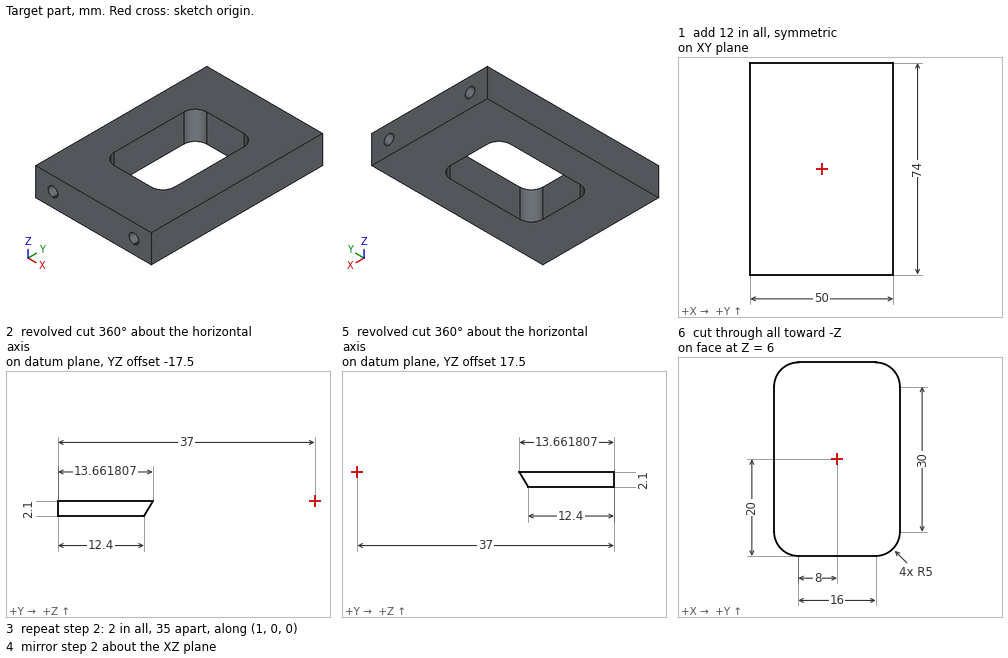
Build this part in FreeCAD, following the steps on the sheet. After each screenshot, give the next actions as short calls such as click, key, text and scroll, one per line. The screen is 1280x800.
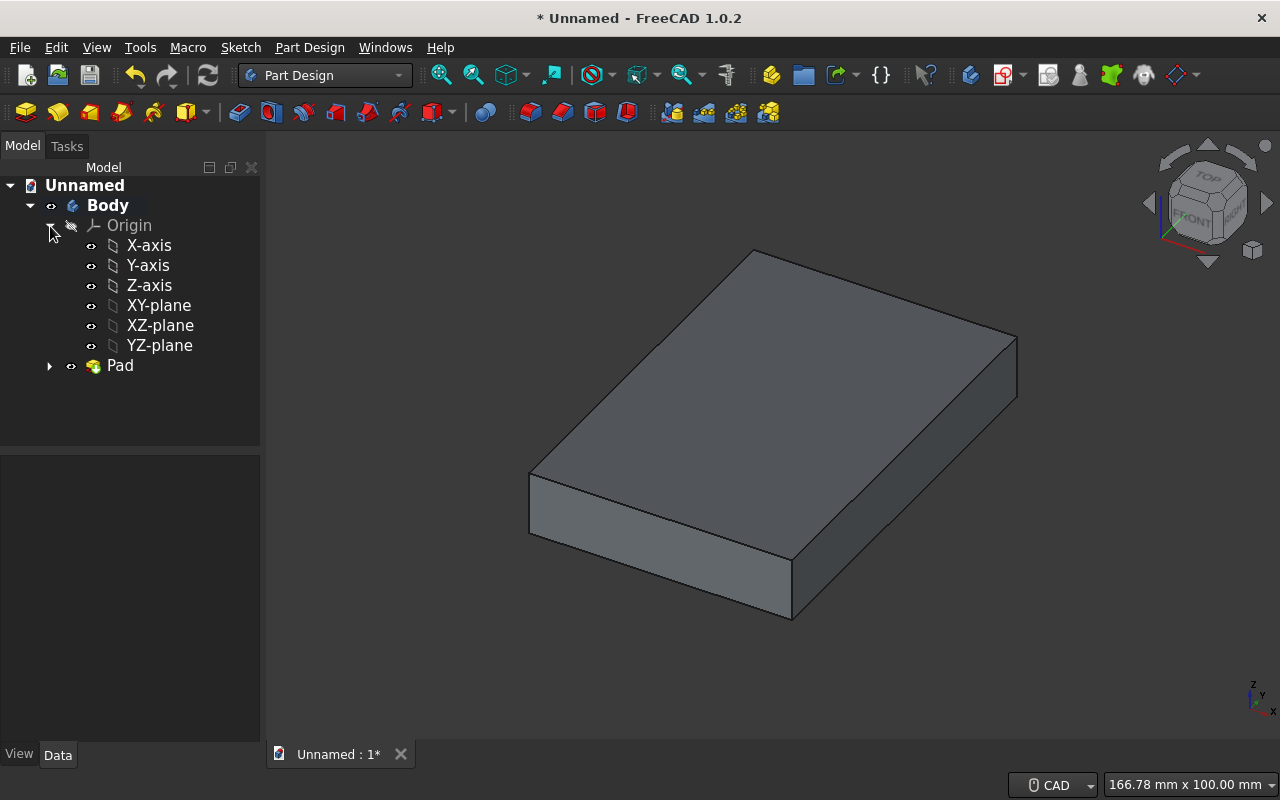
click(136, 346)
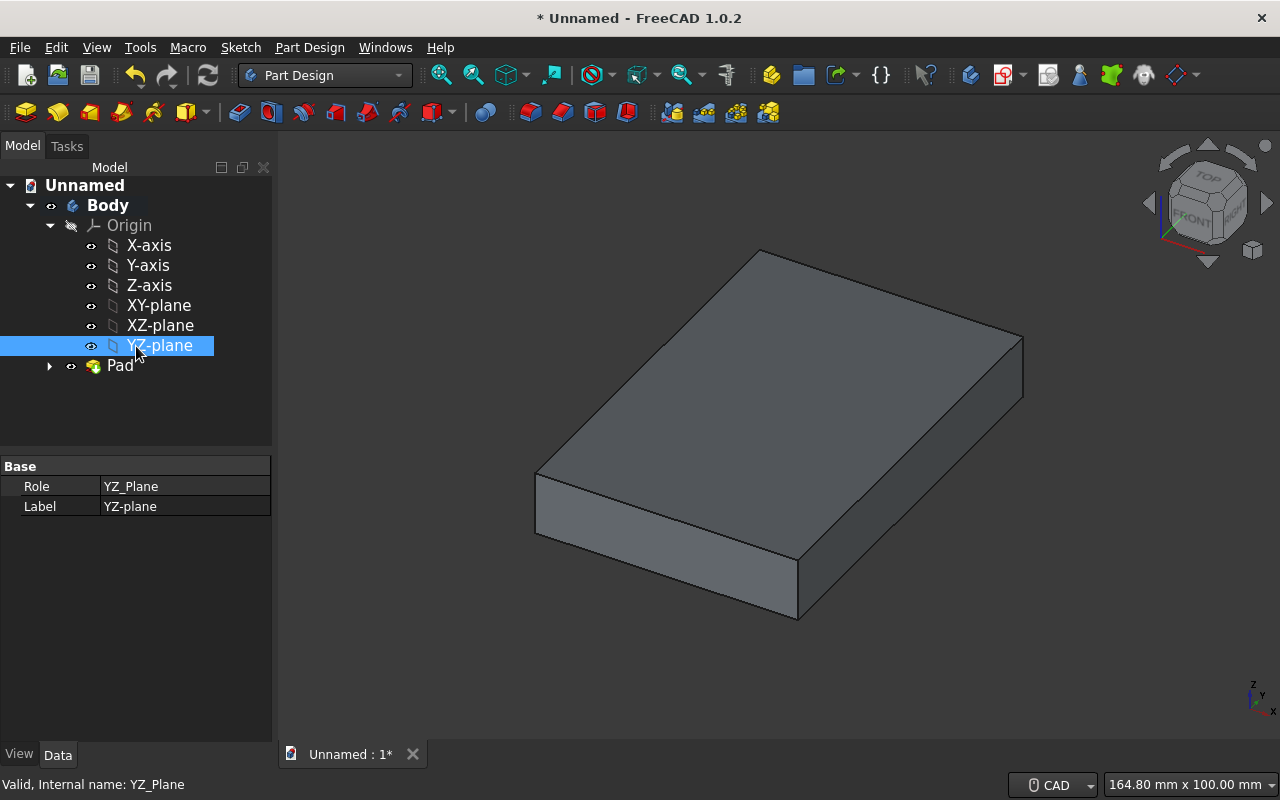
click(1176, 76)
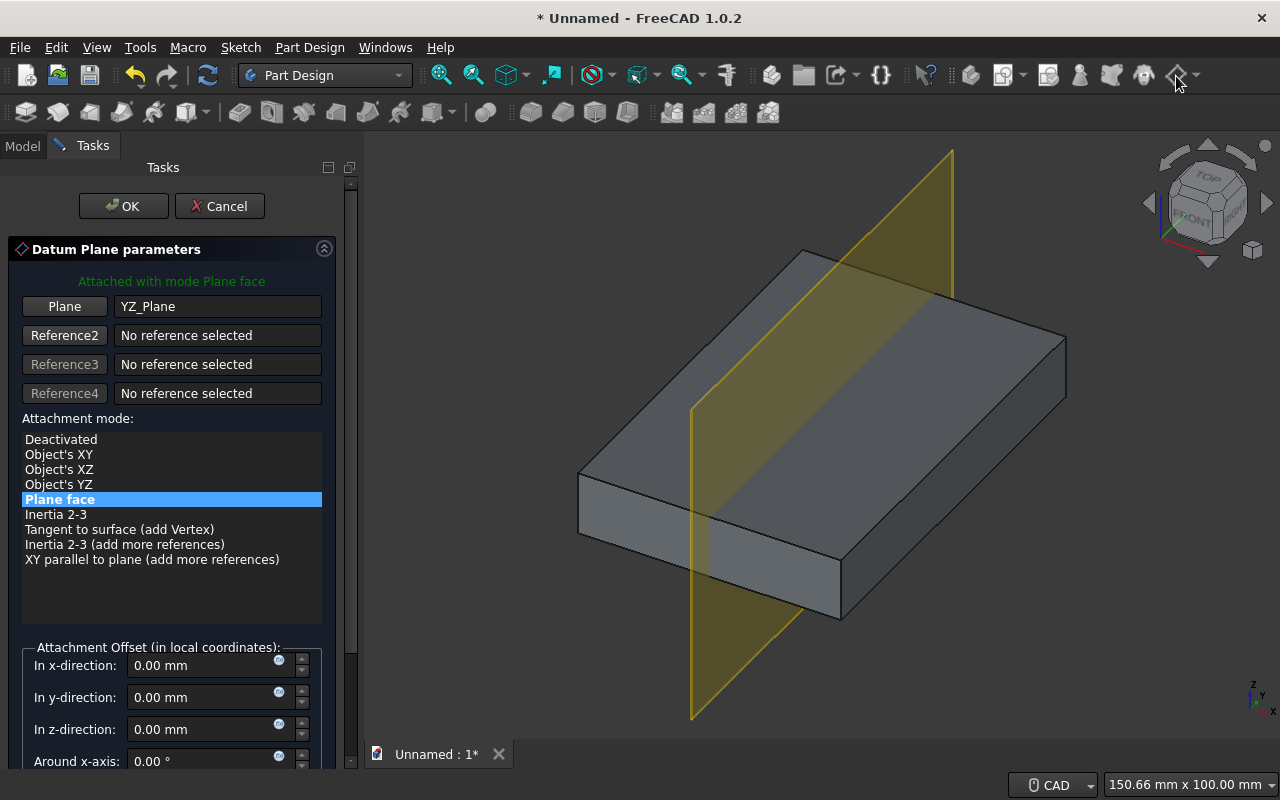
triple_click(210, 729)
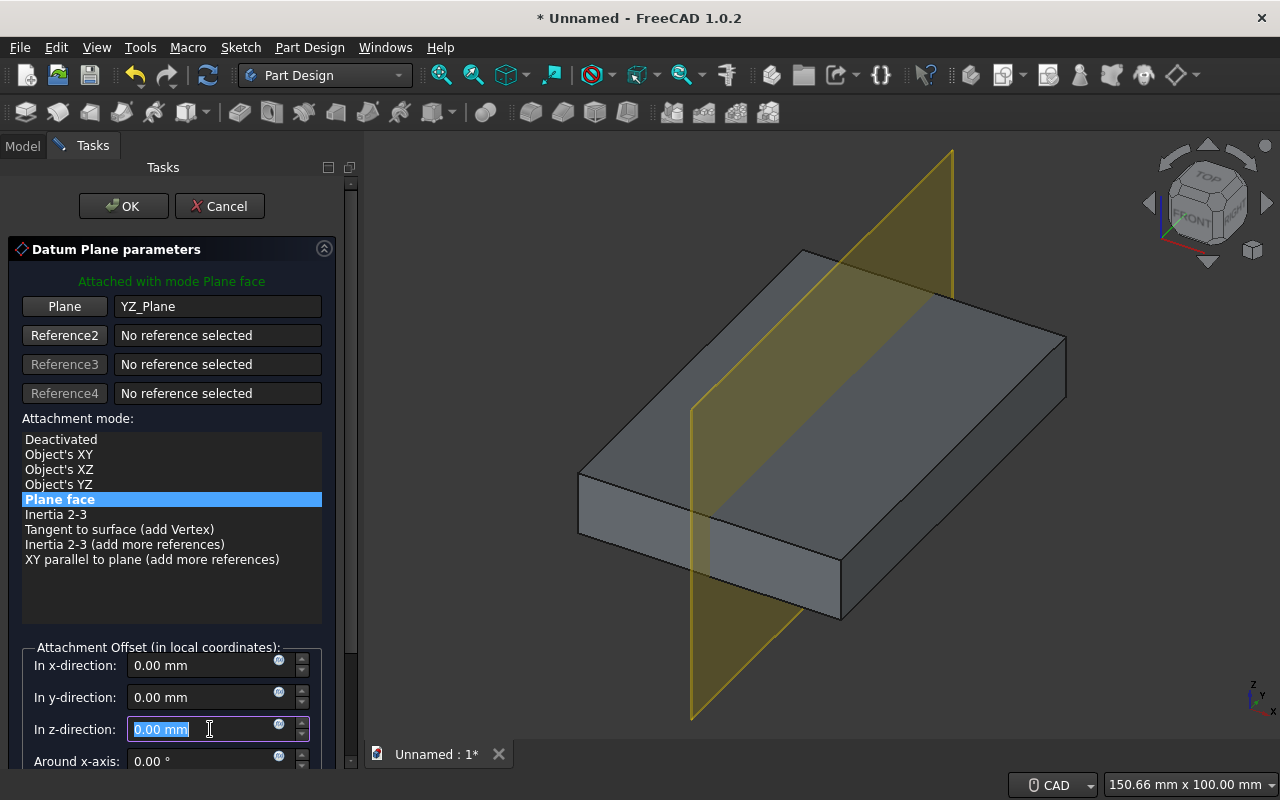
text(-17.5)
key(Tab)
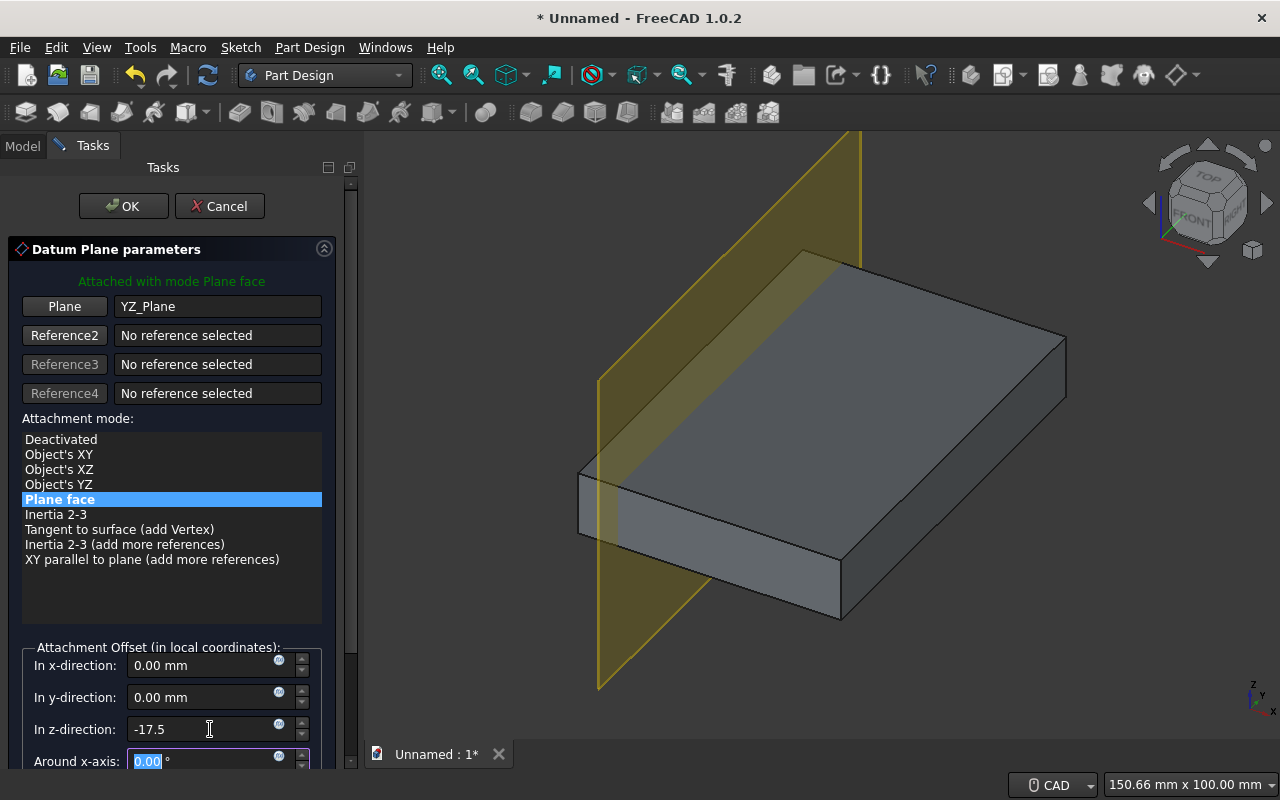
click(124, 206)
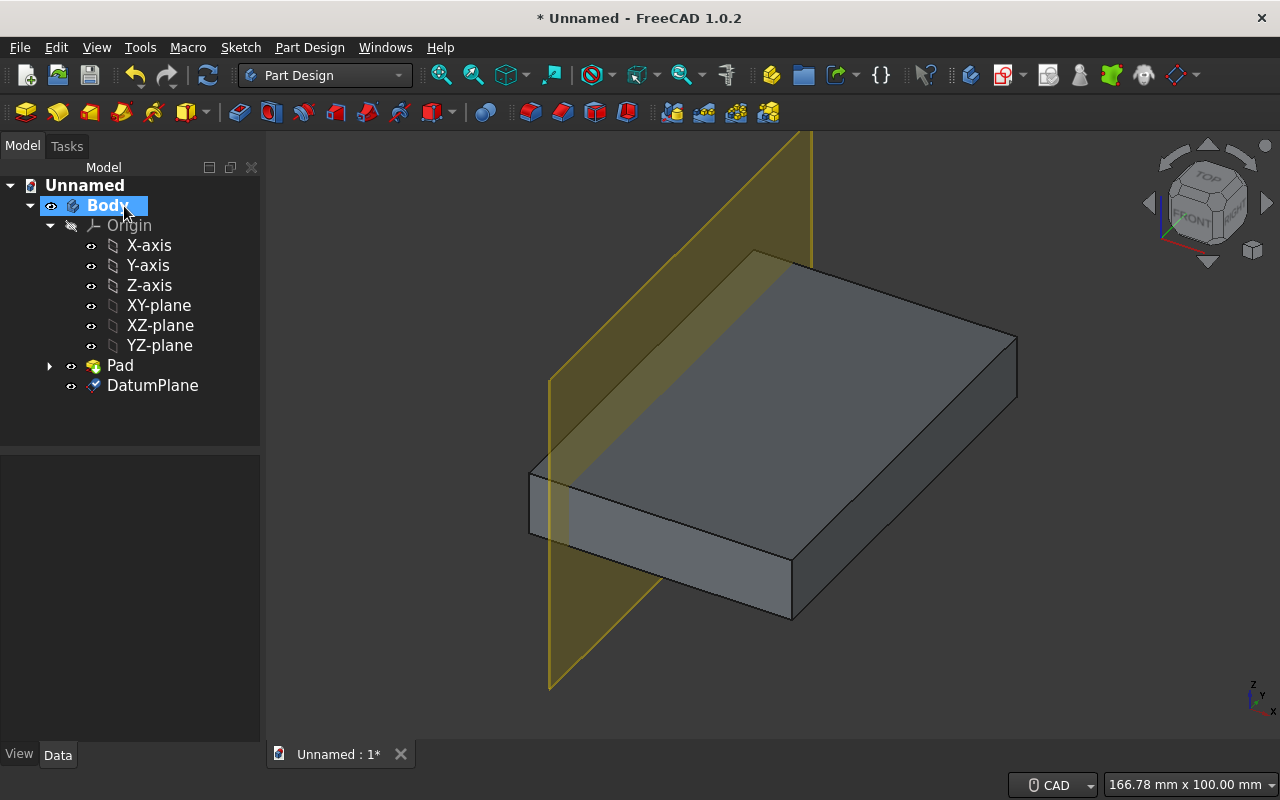
click(116, 386)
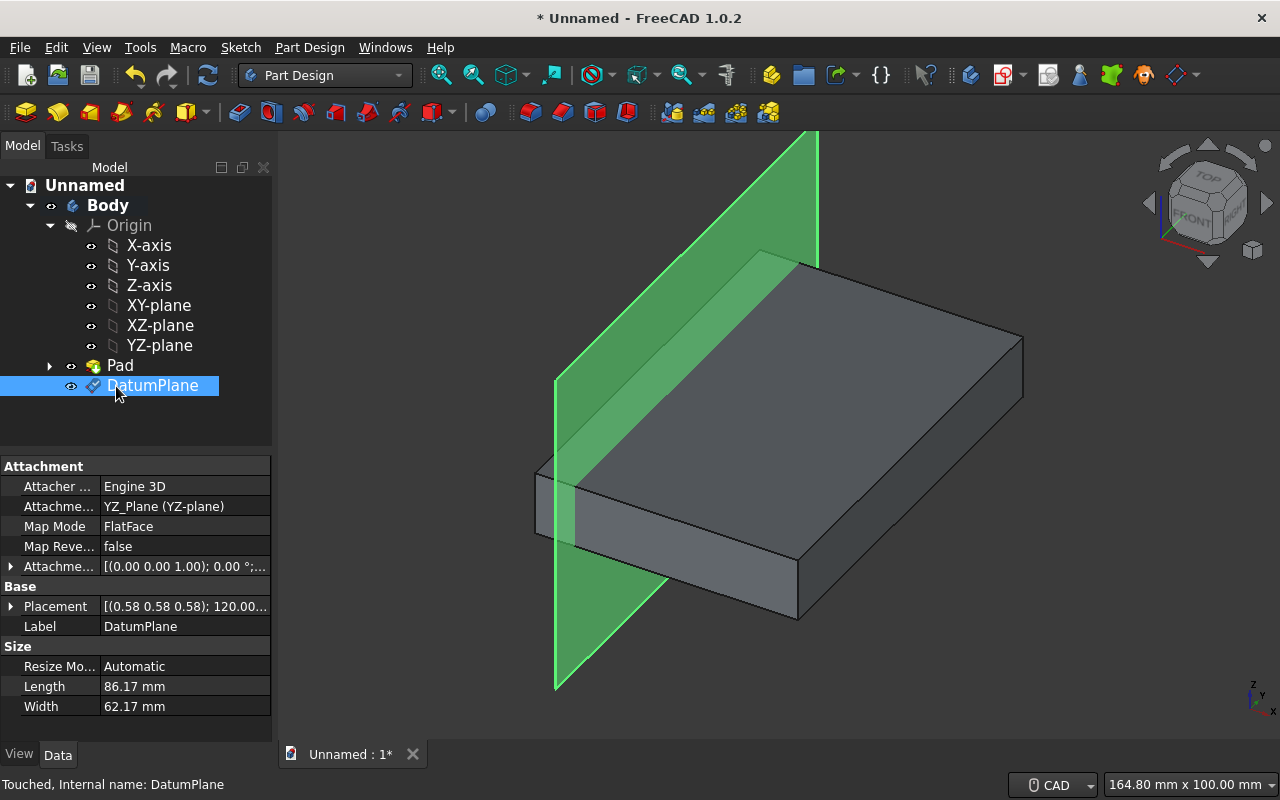
click(1004, 76)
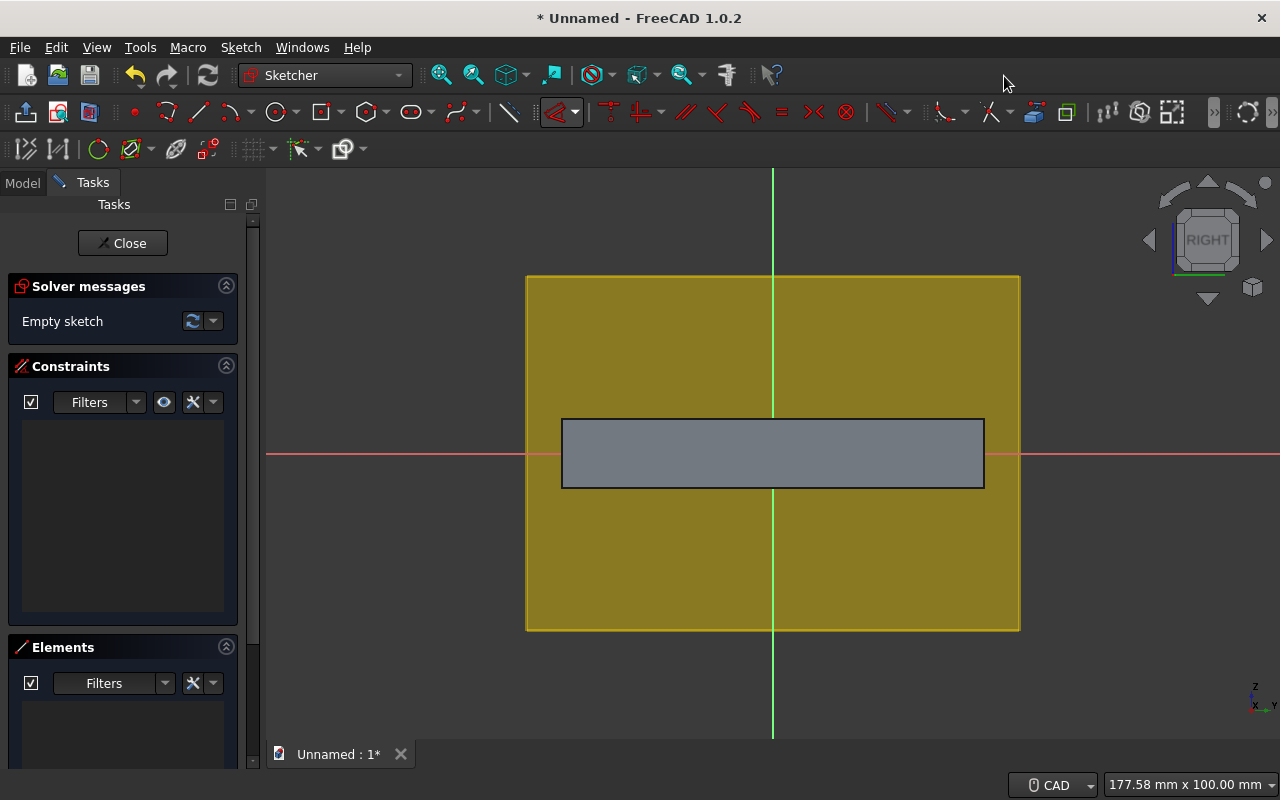
click(90, 112)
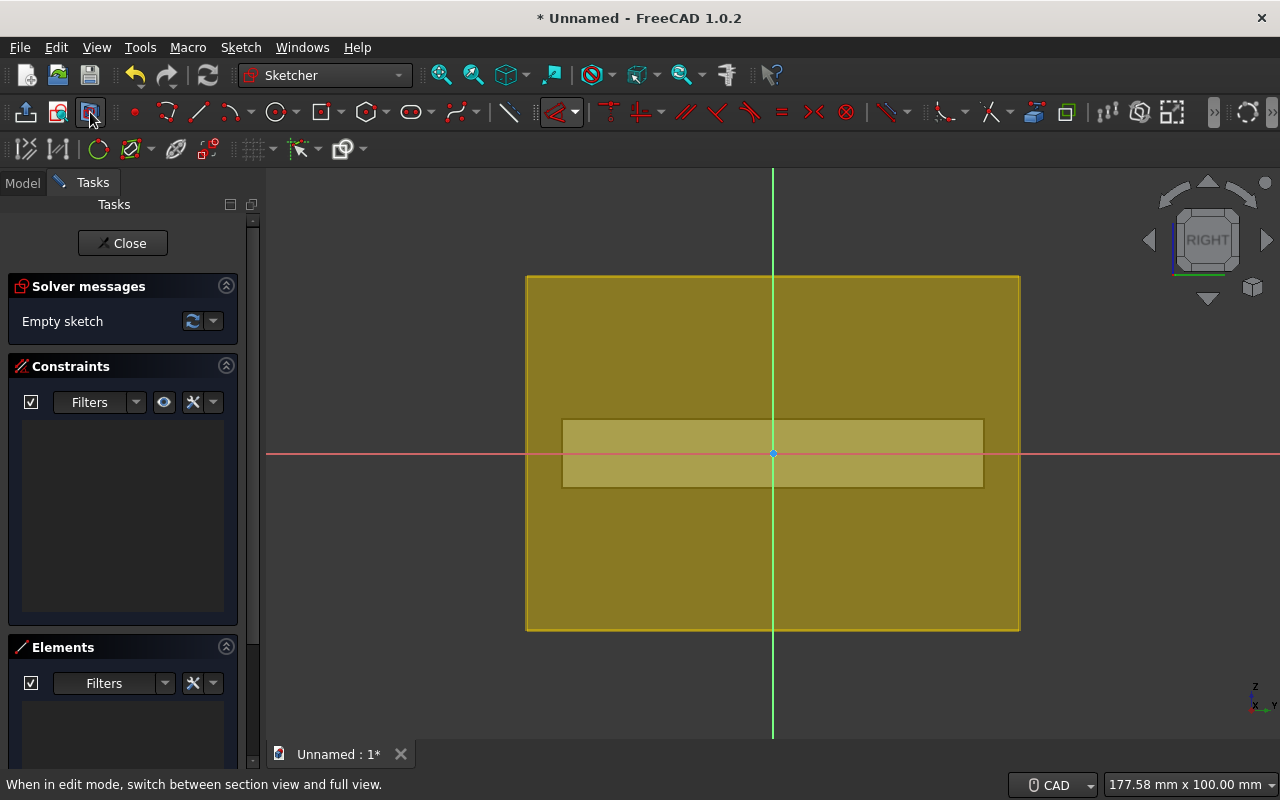
scroll(584, 460, up, 10)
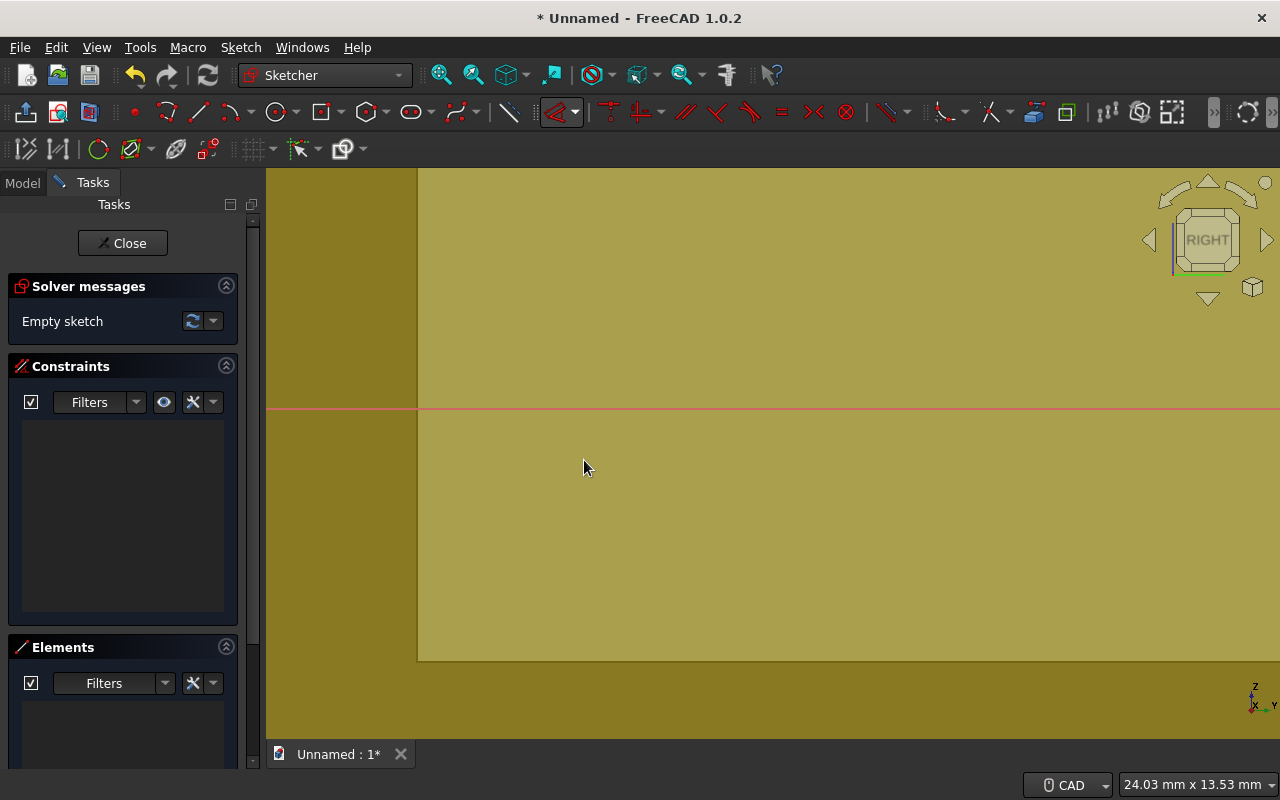
click(168, 112)